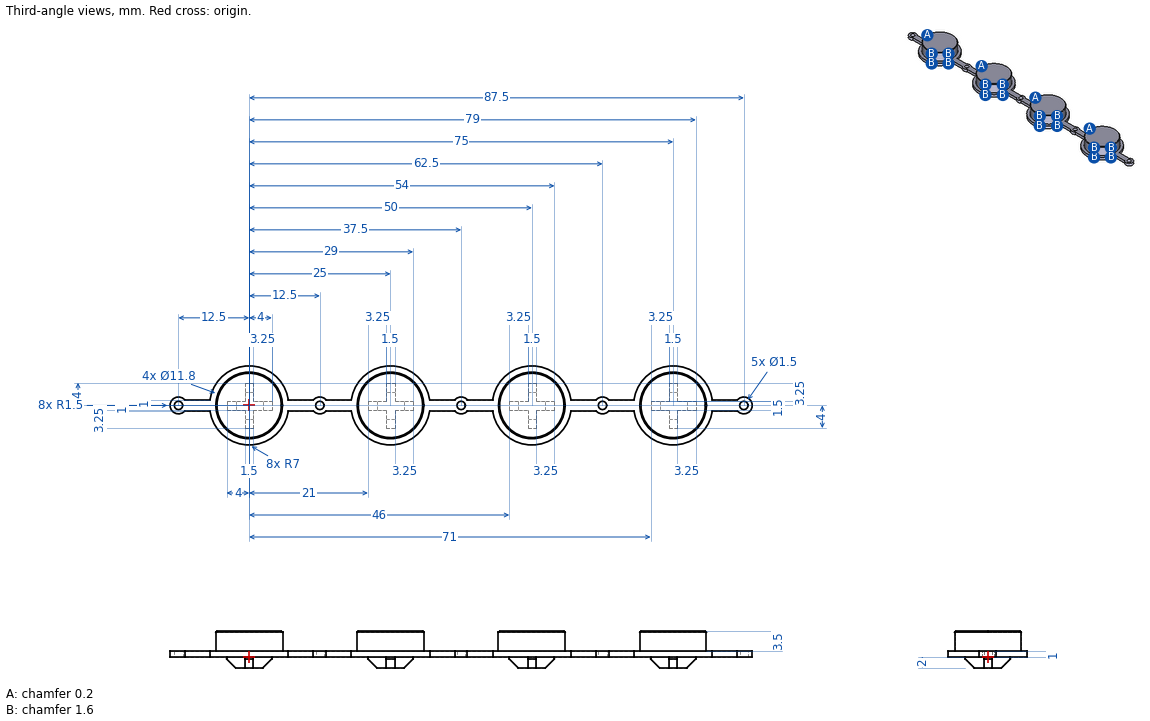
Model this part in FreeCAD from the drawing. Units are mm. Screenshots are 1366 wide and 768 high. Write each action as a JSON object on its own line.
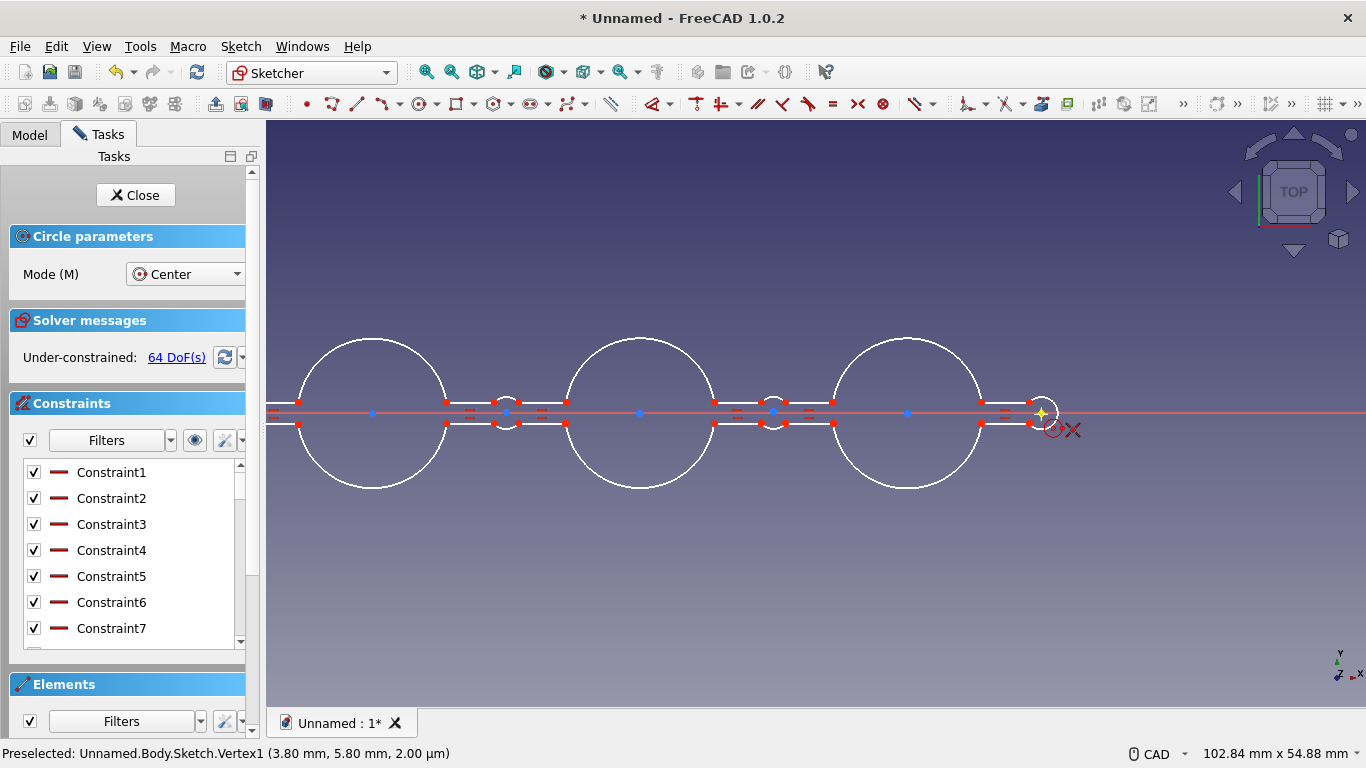
{"action": "left_click", "coordinate": [1041, 413]}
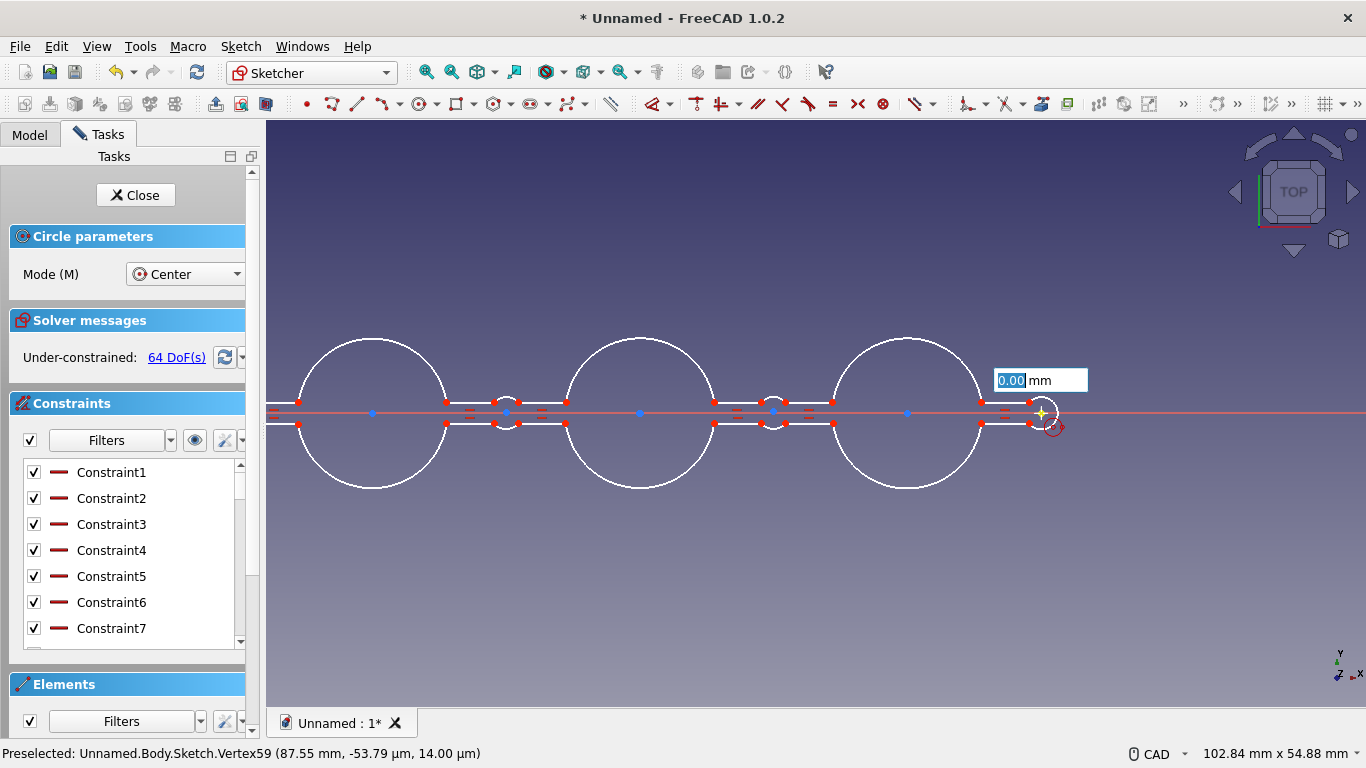
{"action": "scroll", "coordinate": [1038, 420], "scroll_direction": "up", "scroll_amount": 4}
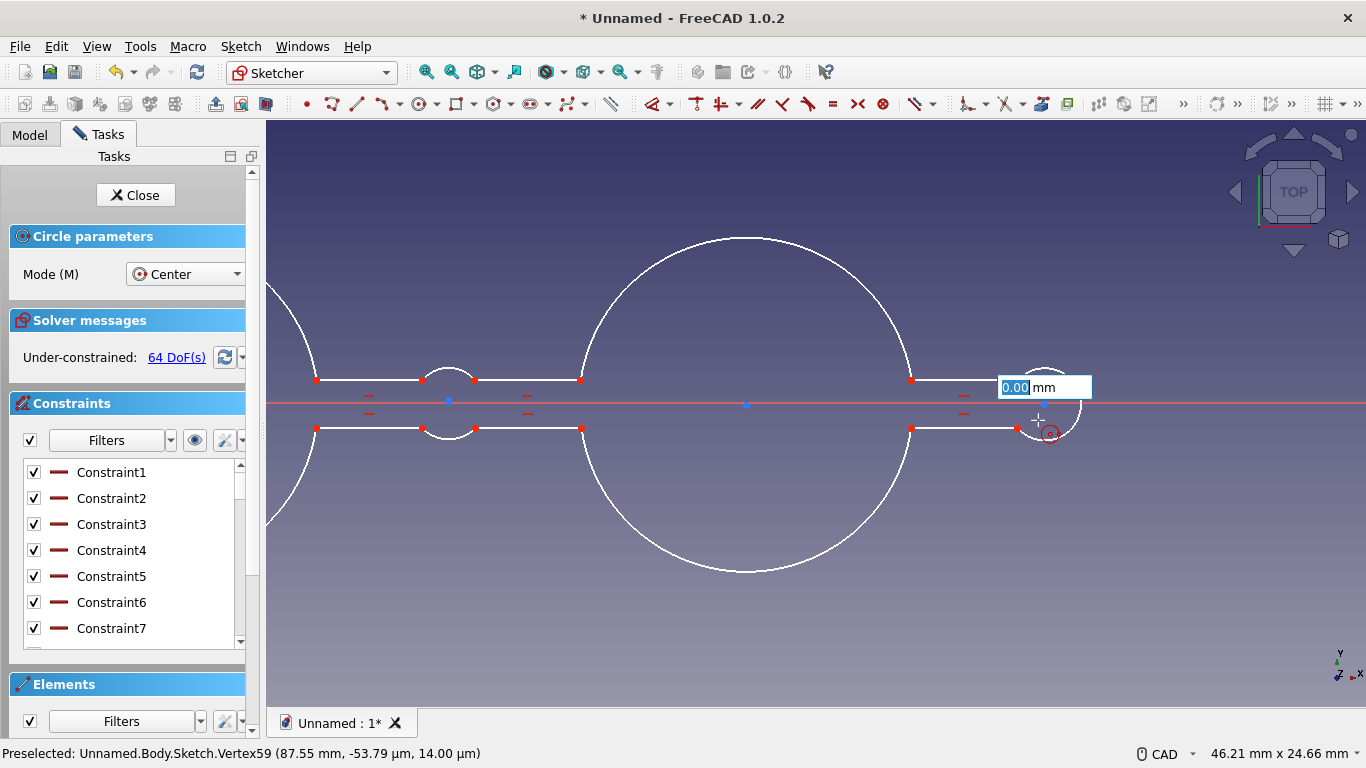
{"action": "left_click", "coordinate": [1038, 420]}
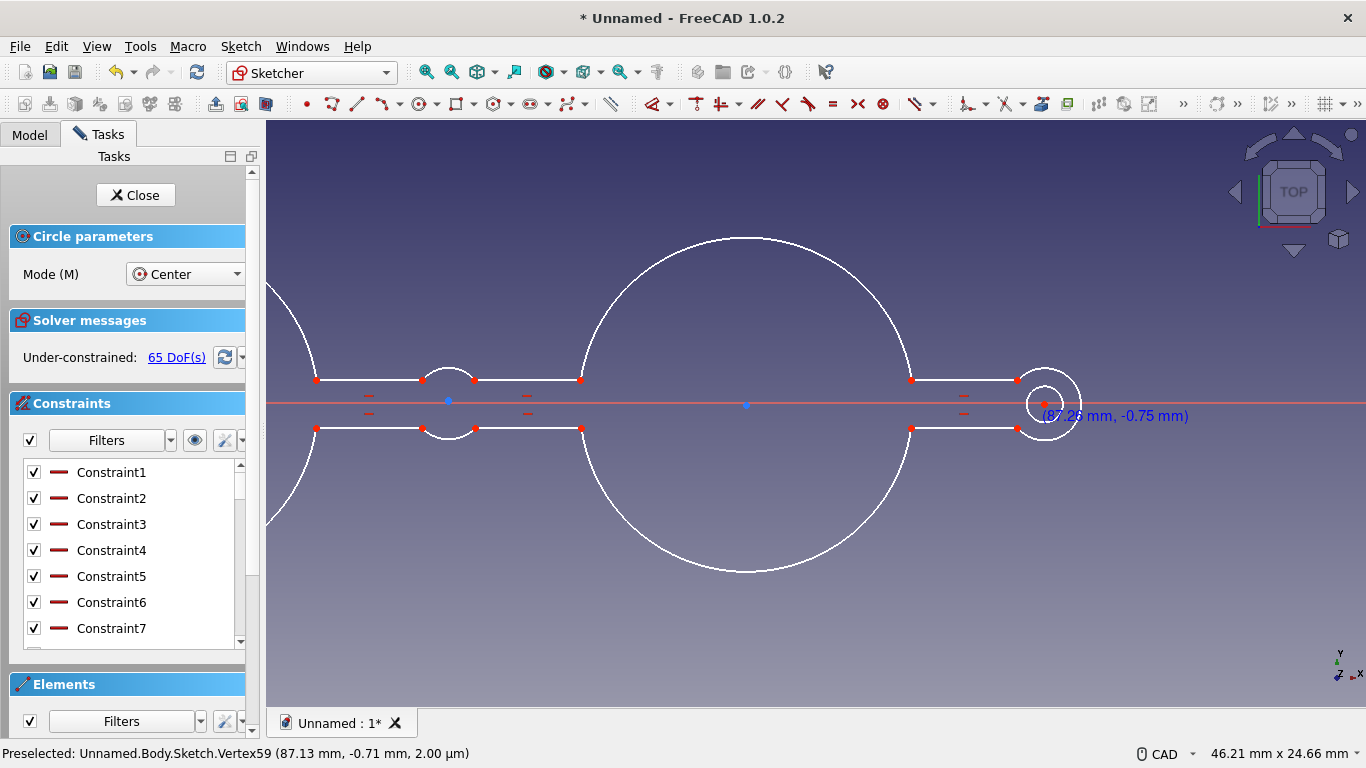
{"action": "scroll", "coordinate": [449, 403], "scroll_direction": "up", "scroll_amount": 2}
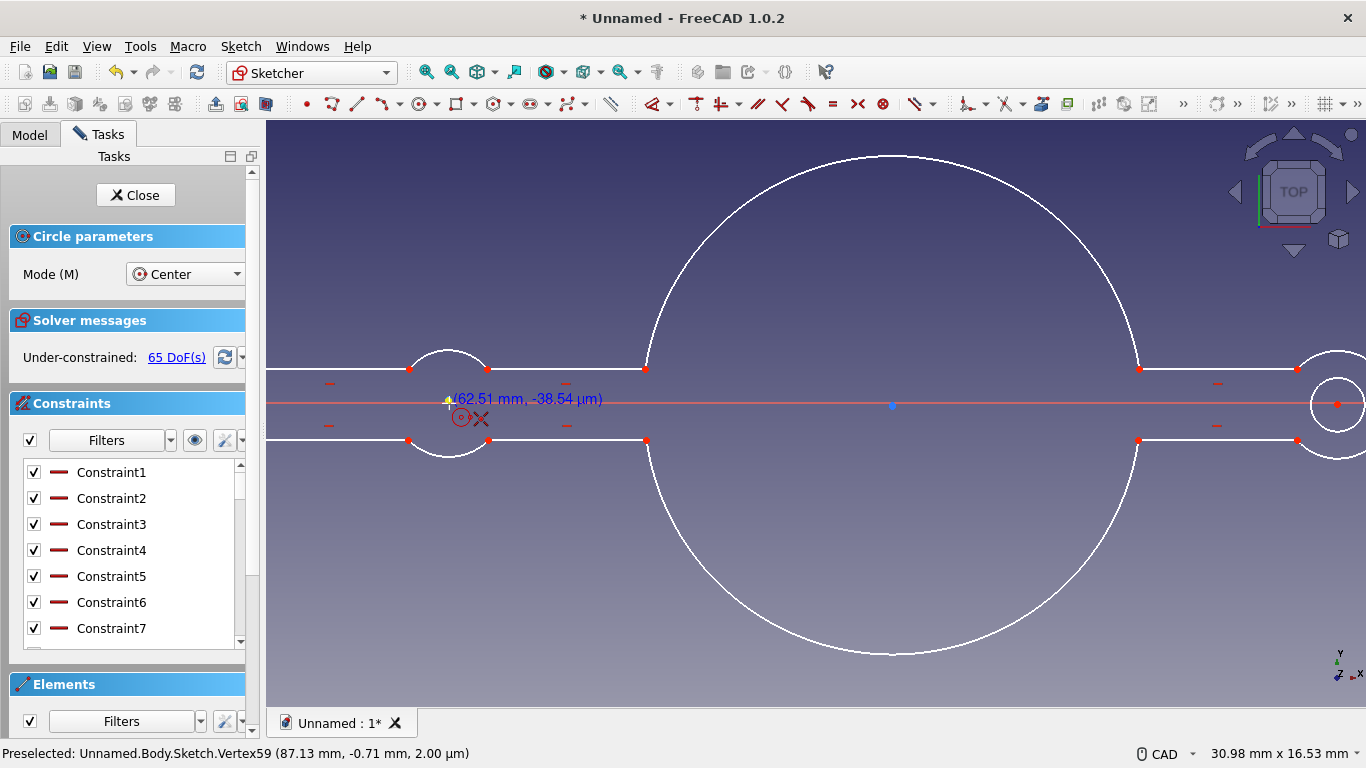
{"action": "scroll", "coordinate": [983, 416], "scroll_direction": "down", "scroll_amount": 9}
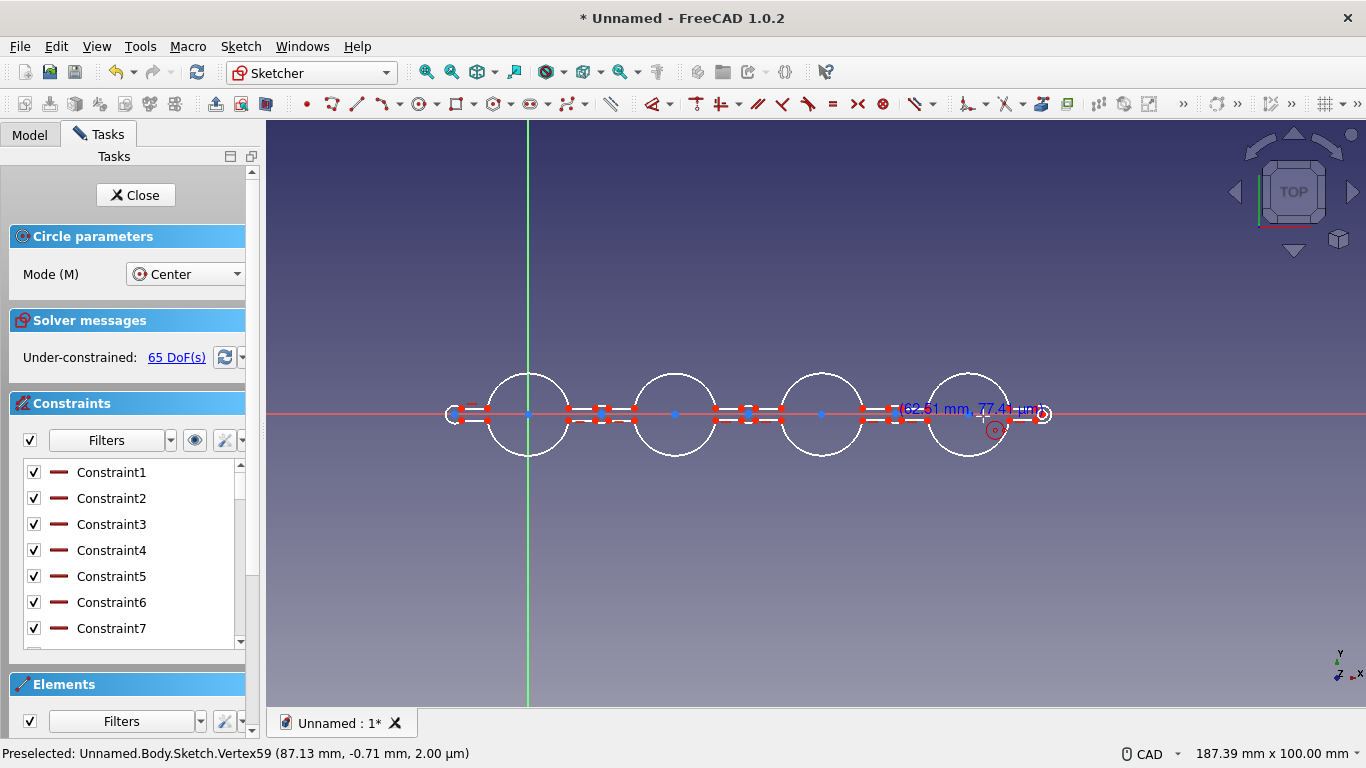
{"action": "scroll", "coordinate": [895, 414], "scroll_direction": "up", "scroll_amount": 3}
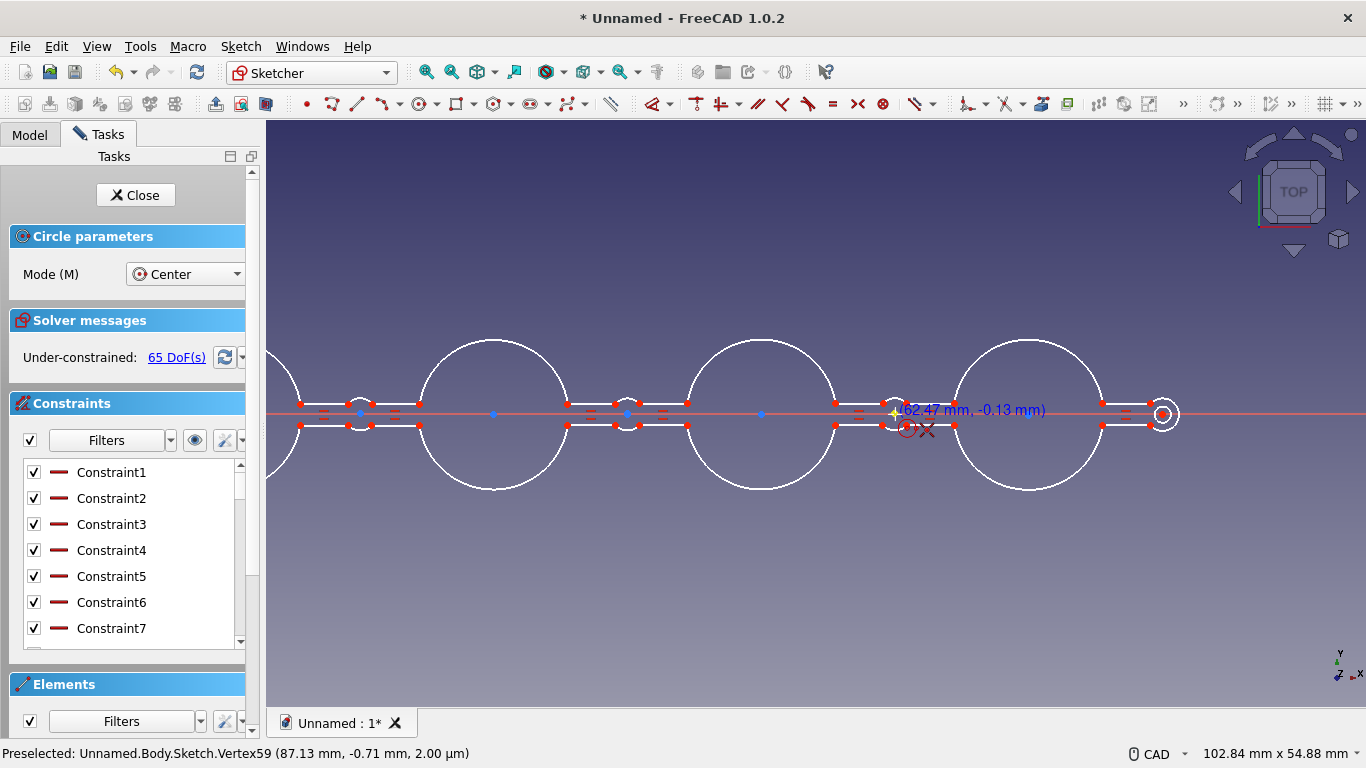
{"action": "left_click", "coordinate": [895, 414]}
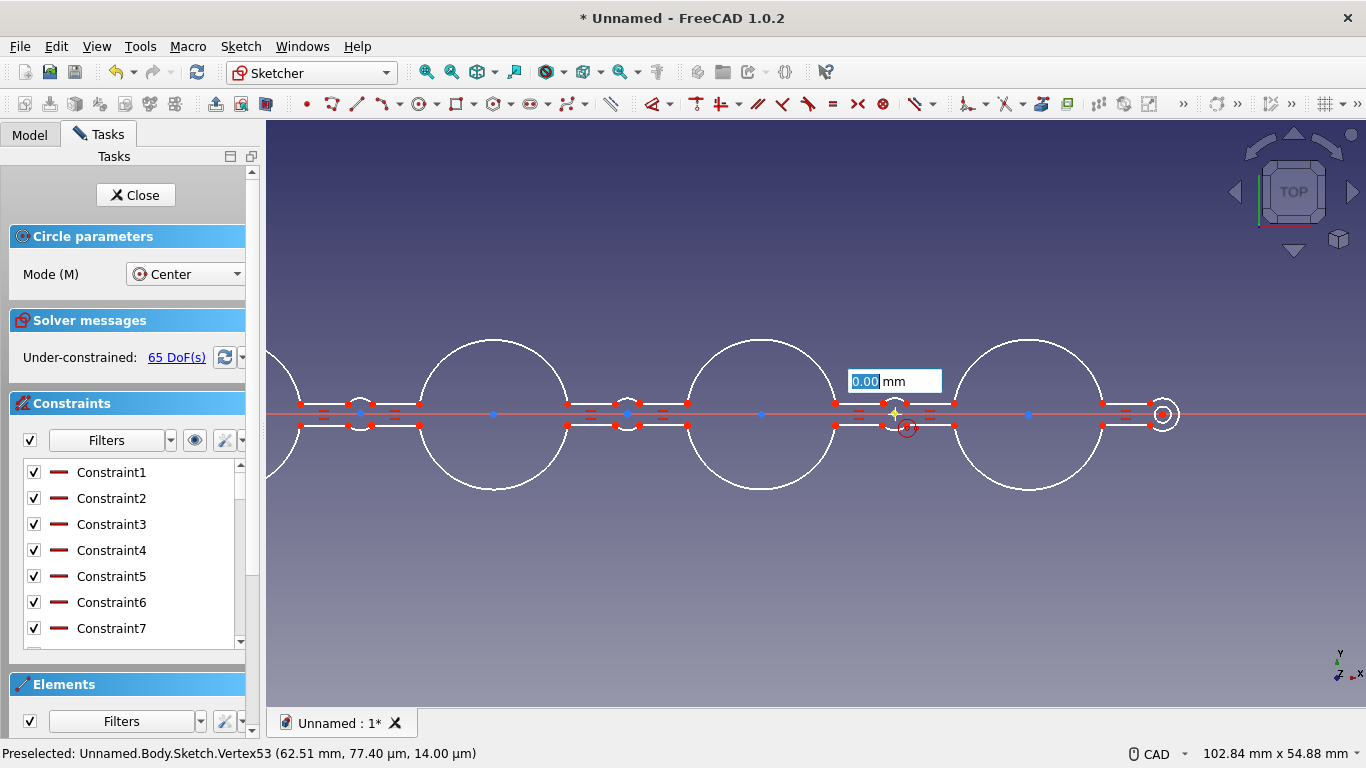
{"action": "scroll", "coordinate": [892, 422], "scroll_direction": "up", "scroll_amount": 4}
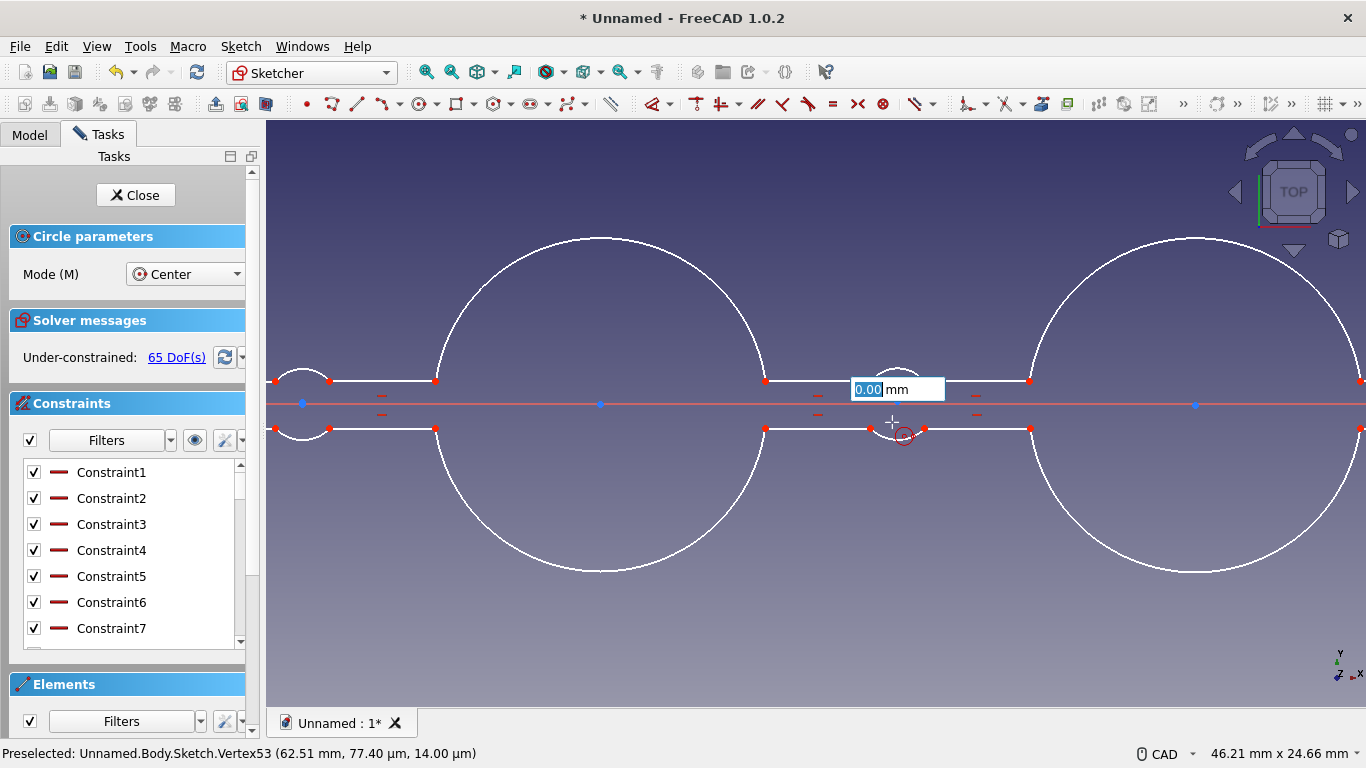
{"action": "left_click", "coordinate": [892, 420]}